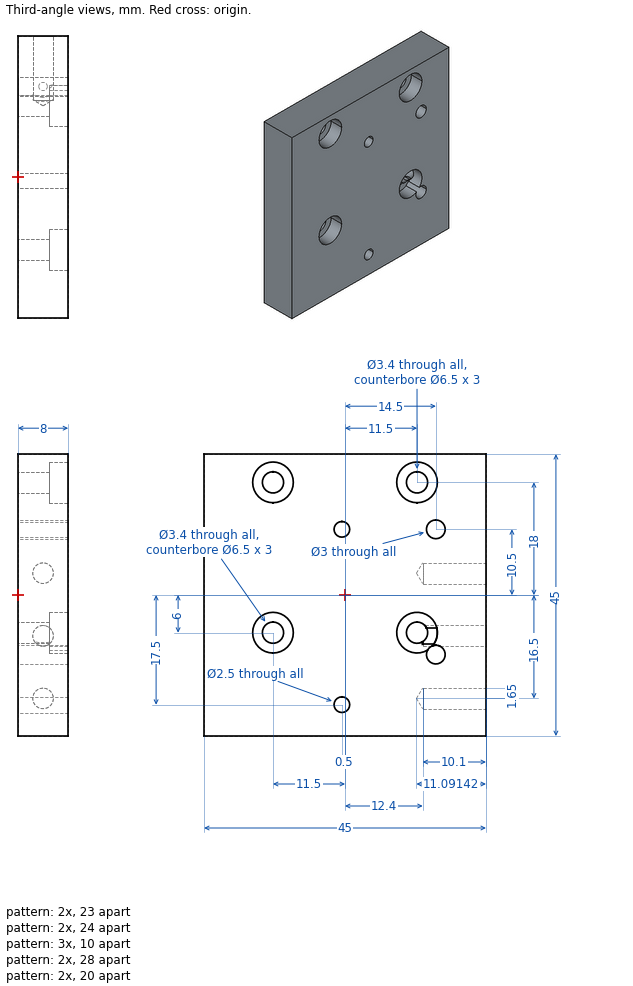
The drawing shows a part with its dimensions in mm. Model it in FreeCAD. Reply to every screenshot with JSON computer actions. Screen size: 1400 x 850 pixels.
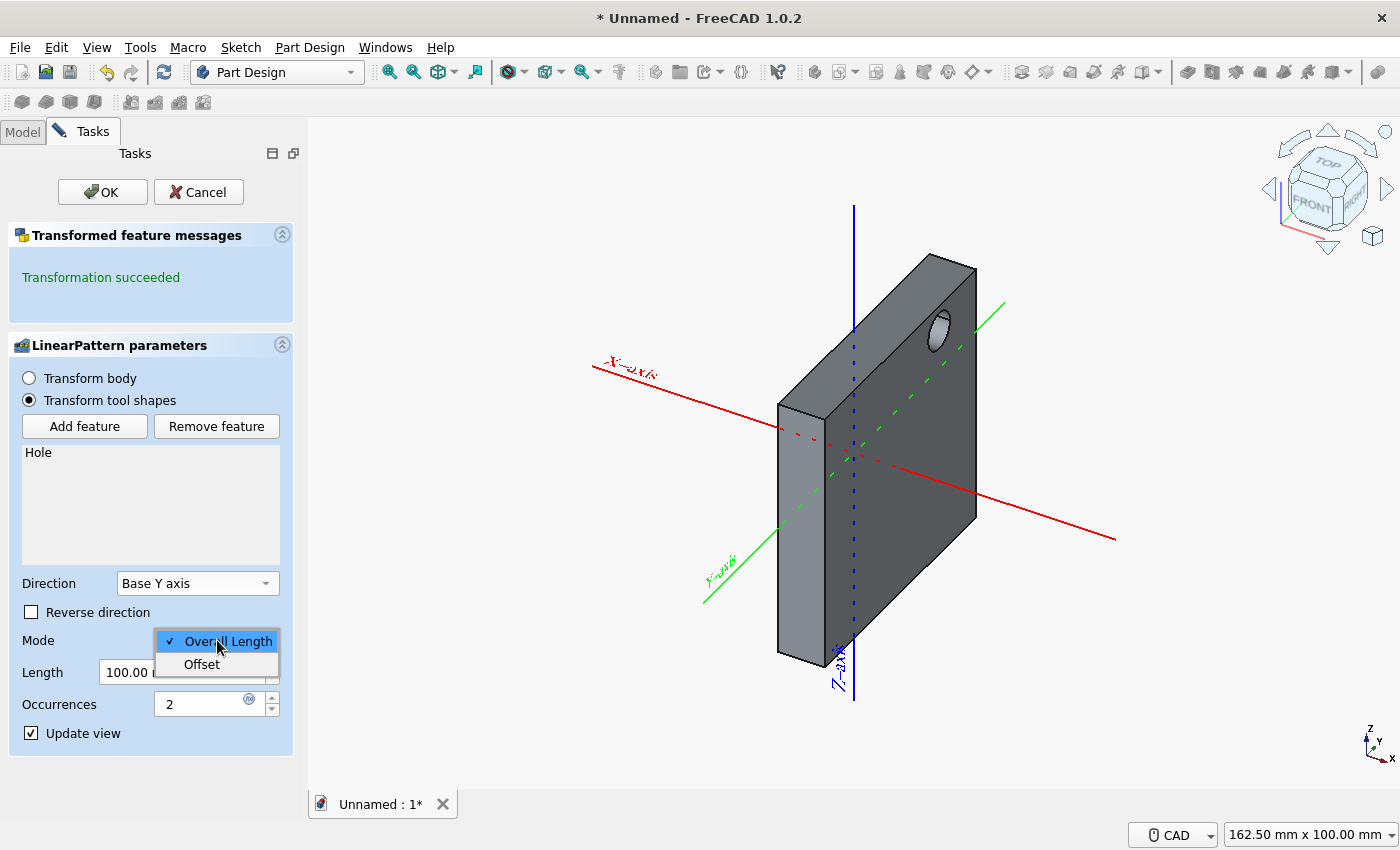
{"action": "left_click", "coordinate": [216, 664]}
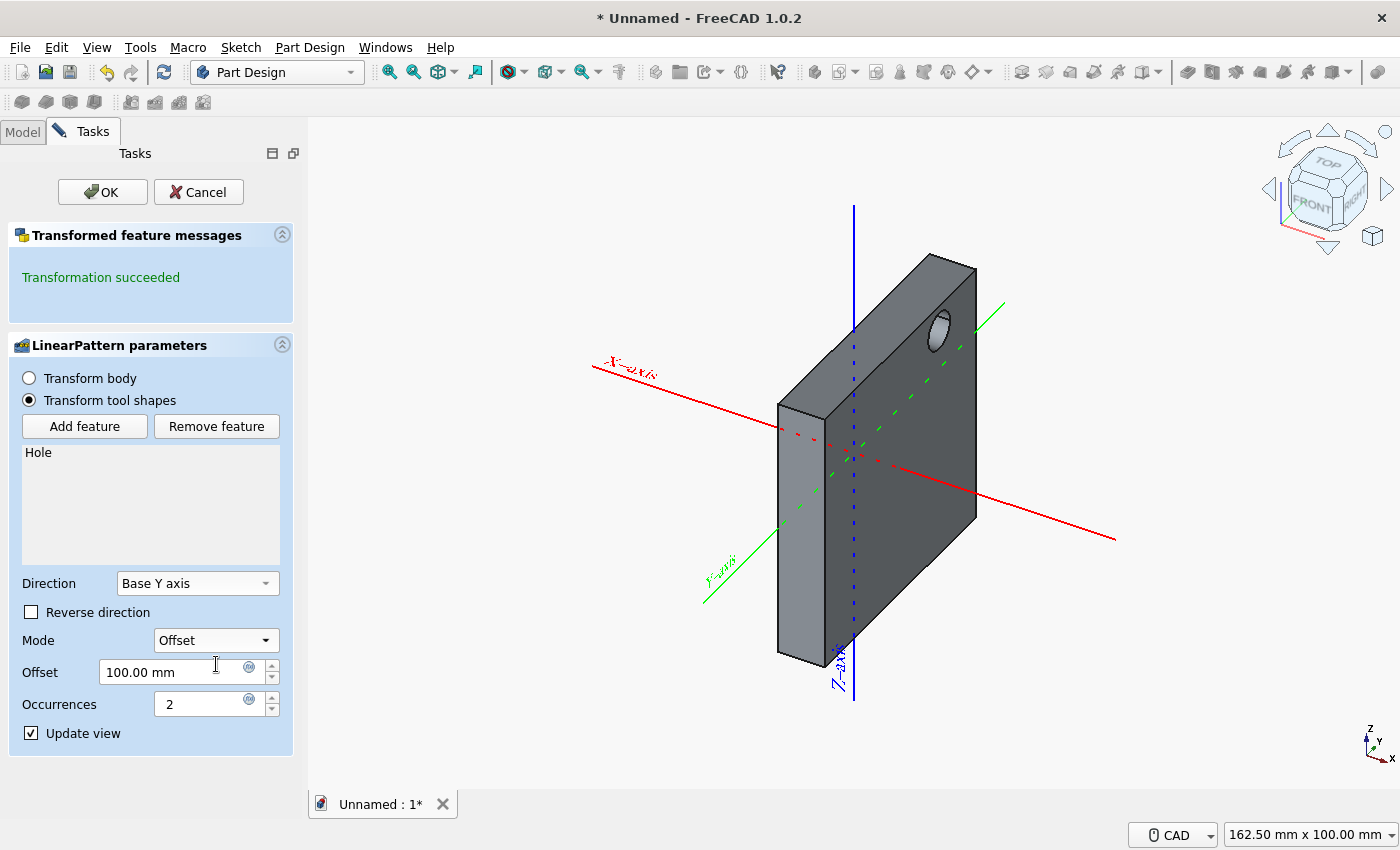
{"action": "triple_click", "coordinate": [182, 672]}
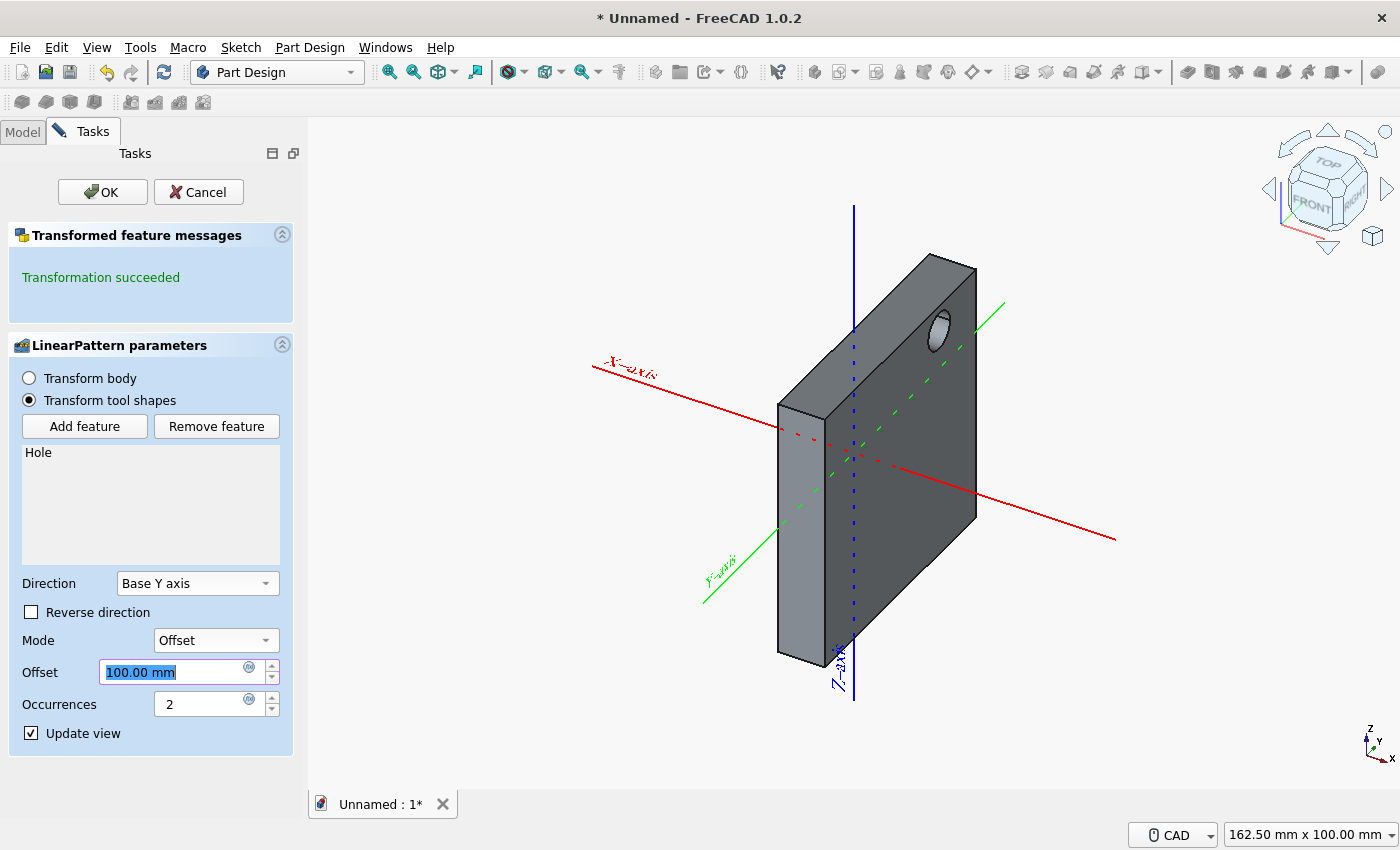
{"action": "type", "text": "23"}
{"action": "key", "text": "Tab"}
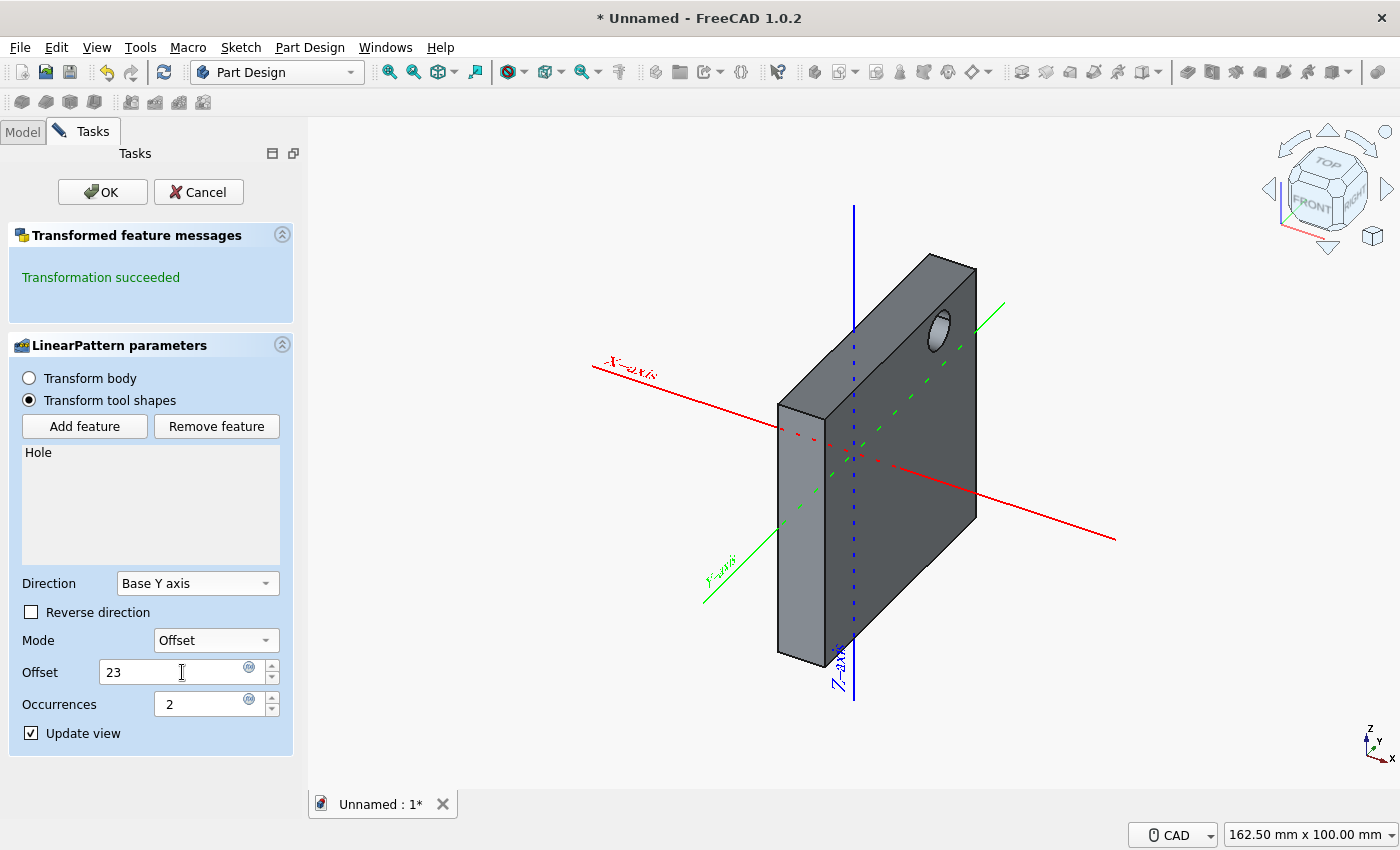
{"action": "triple_click", "coordinate": [209, 704]}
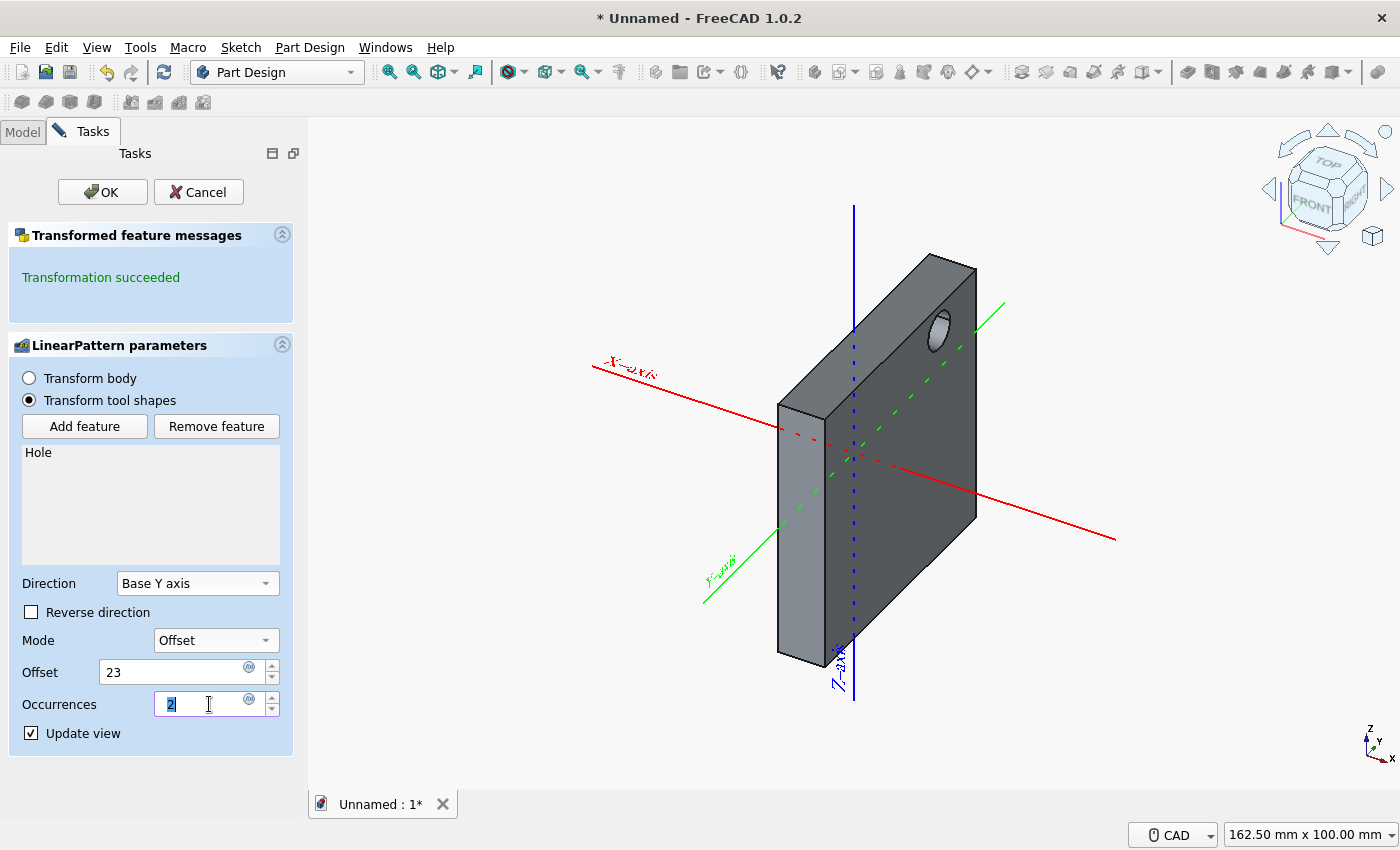
{"action": "type", "text": "2"}
{"action": "key", "text": "Tab"}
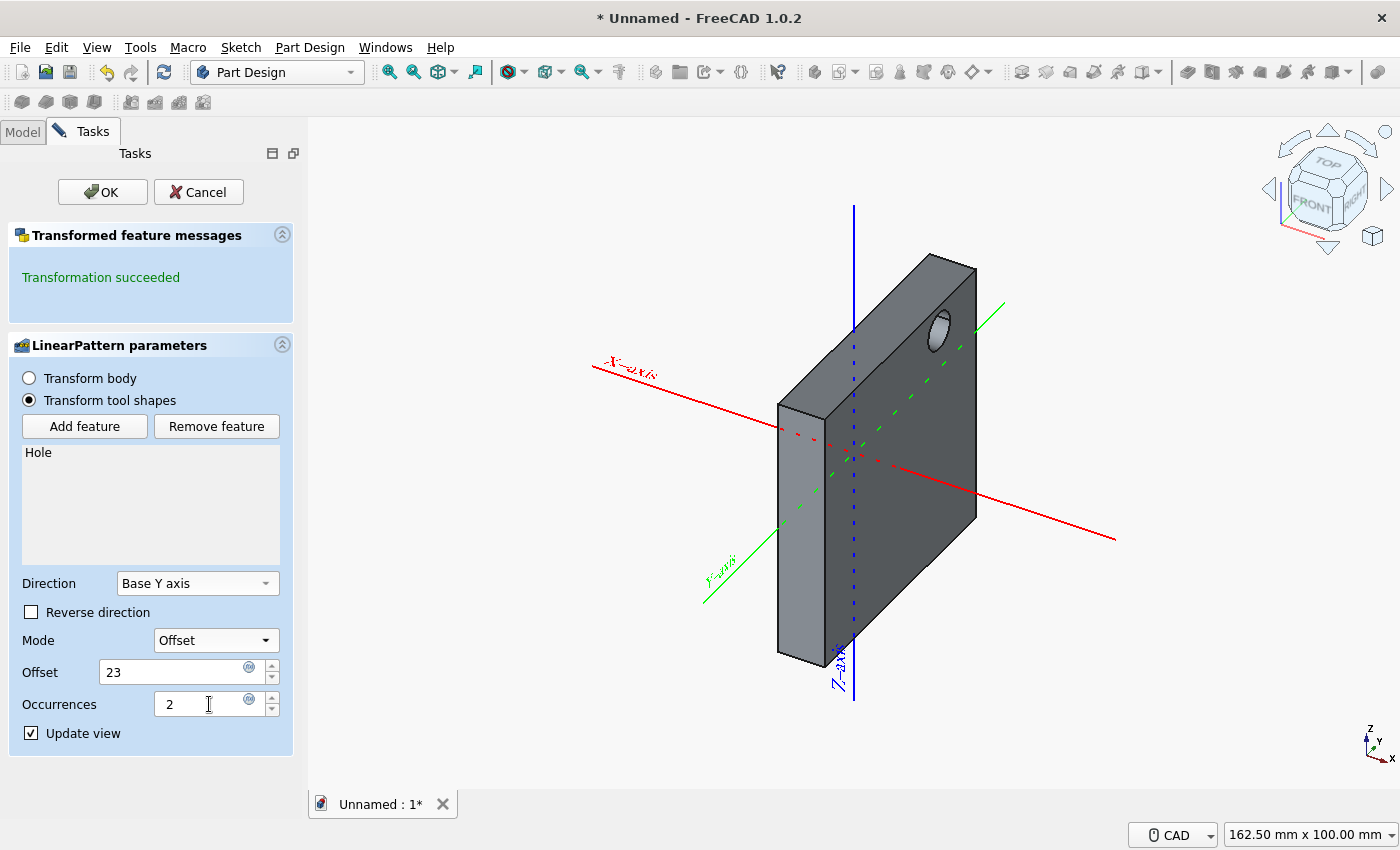
{"action": "left_click", "coordinate": [30, 612]}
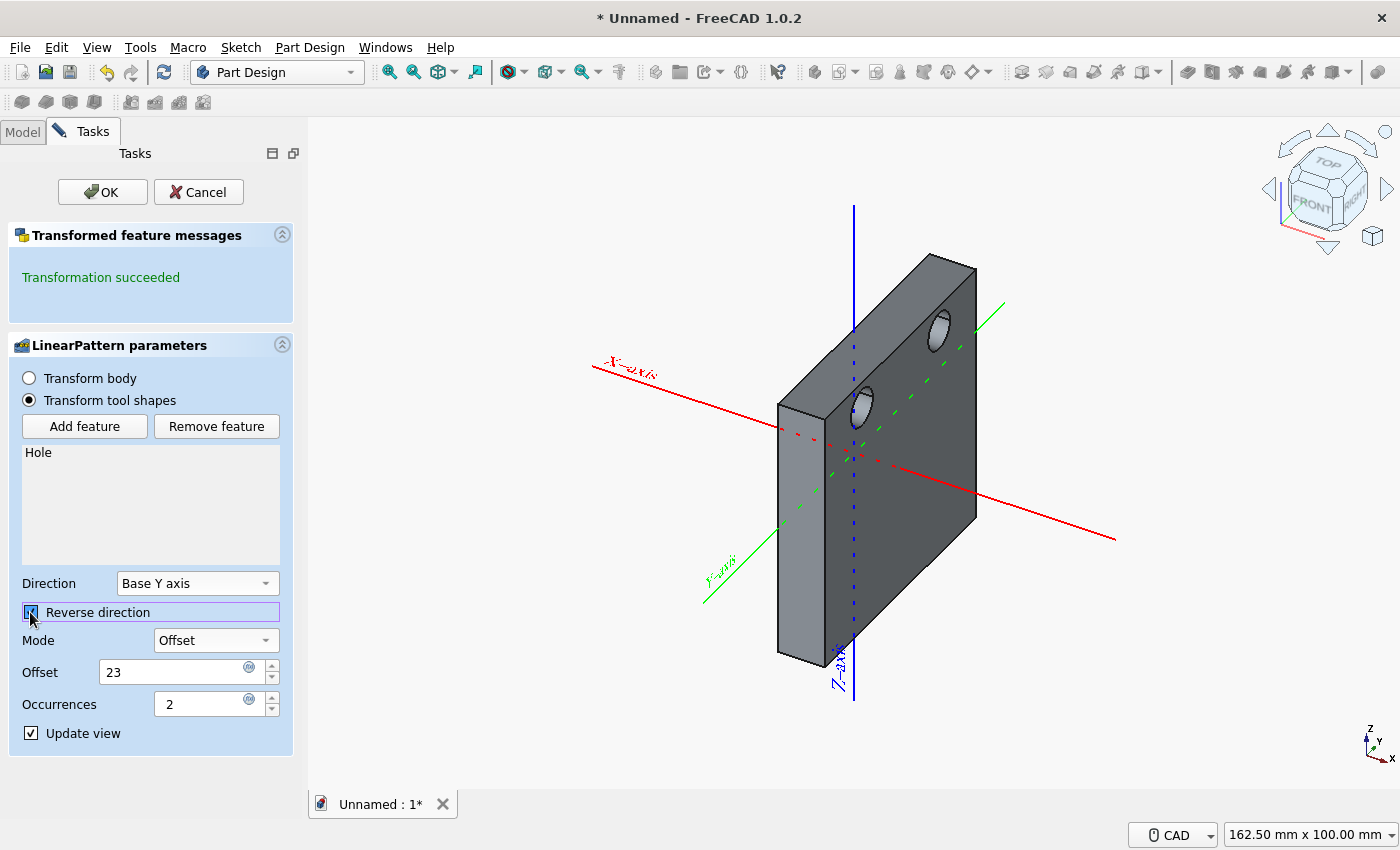
{"action": "left_click", "coordinate": [103, 192]}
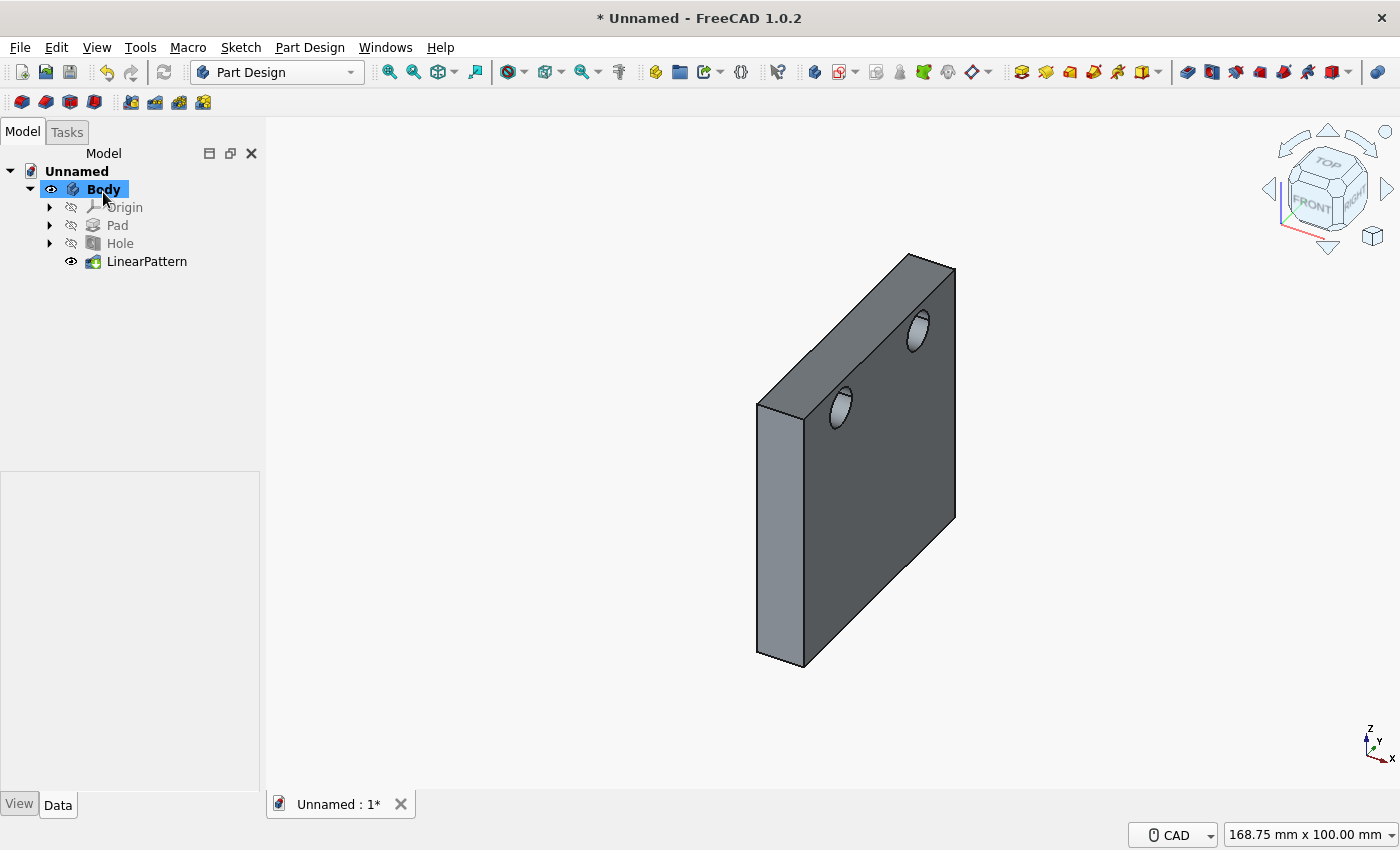
{"action": "left_click", "coordinate": [116, 243]}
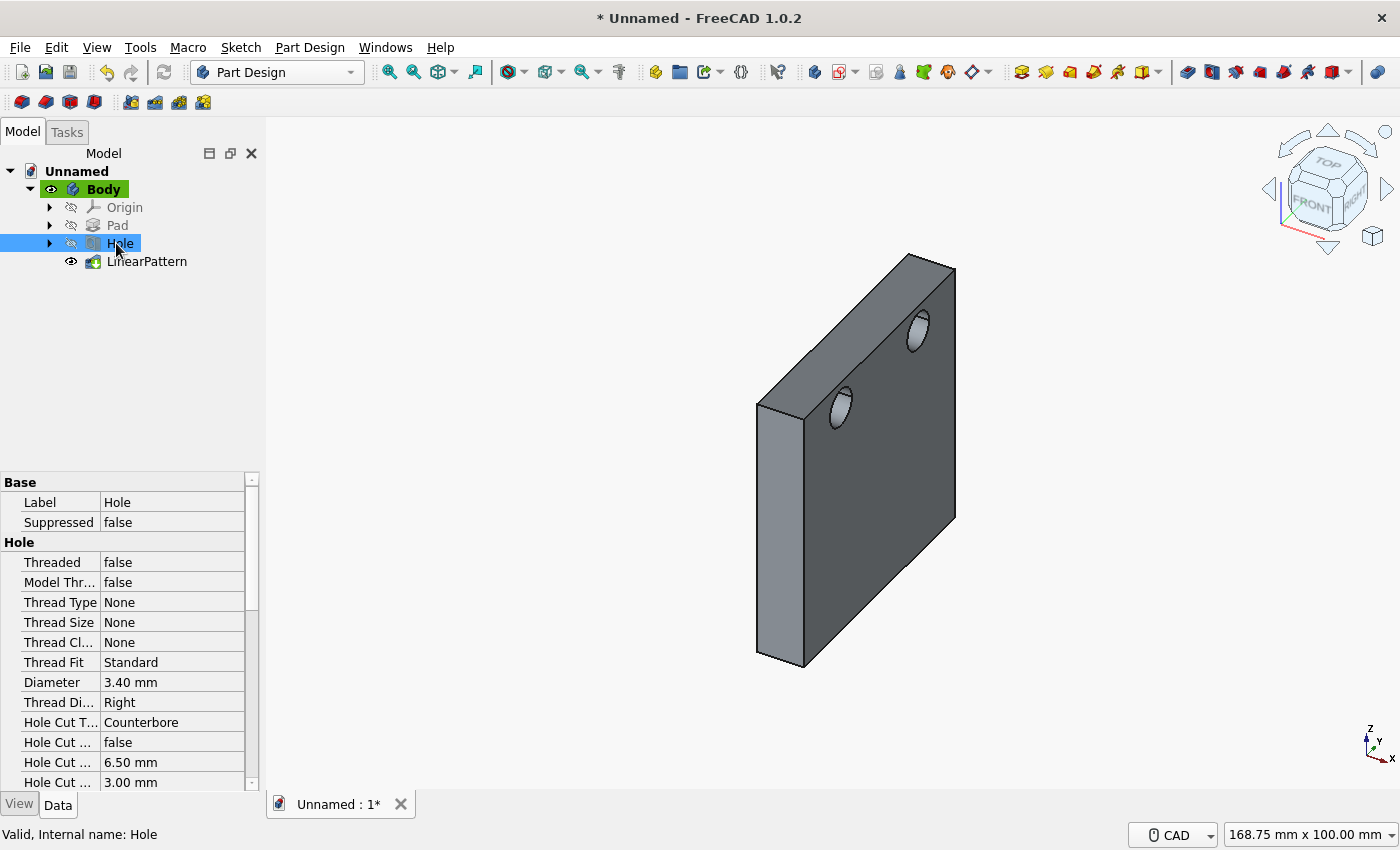
{"action": "left_click", "coordinate": [156, 102]}